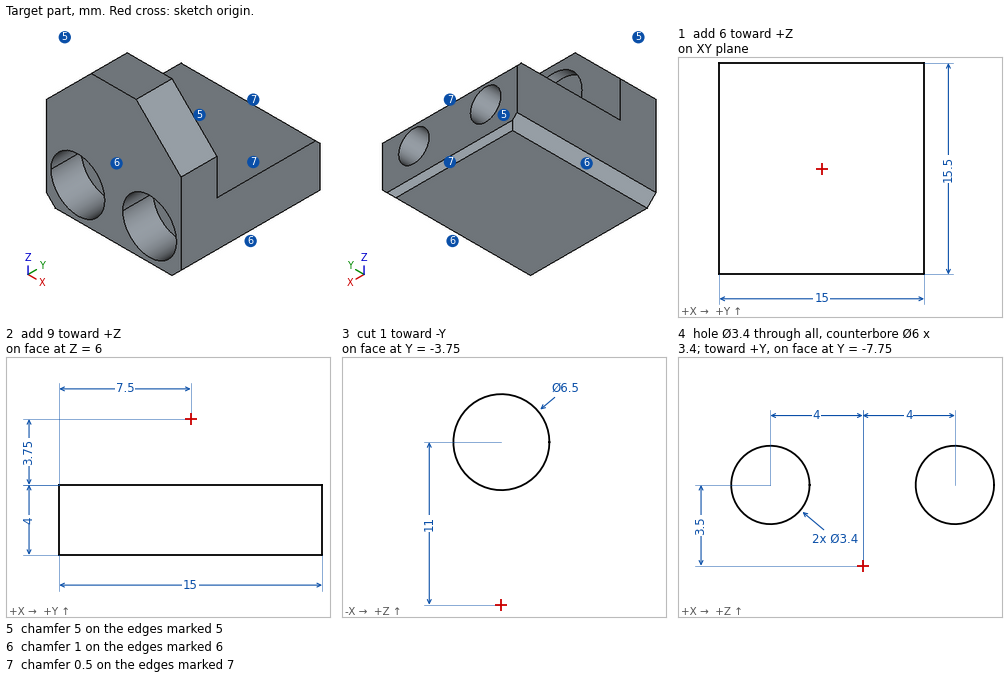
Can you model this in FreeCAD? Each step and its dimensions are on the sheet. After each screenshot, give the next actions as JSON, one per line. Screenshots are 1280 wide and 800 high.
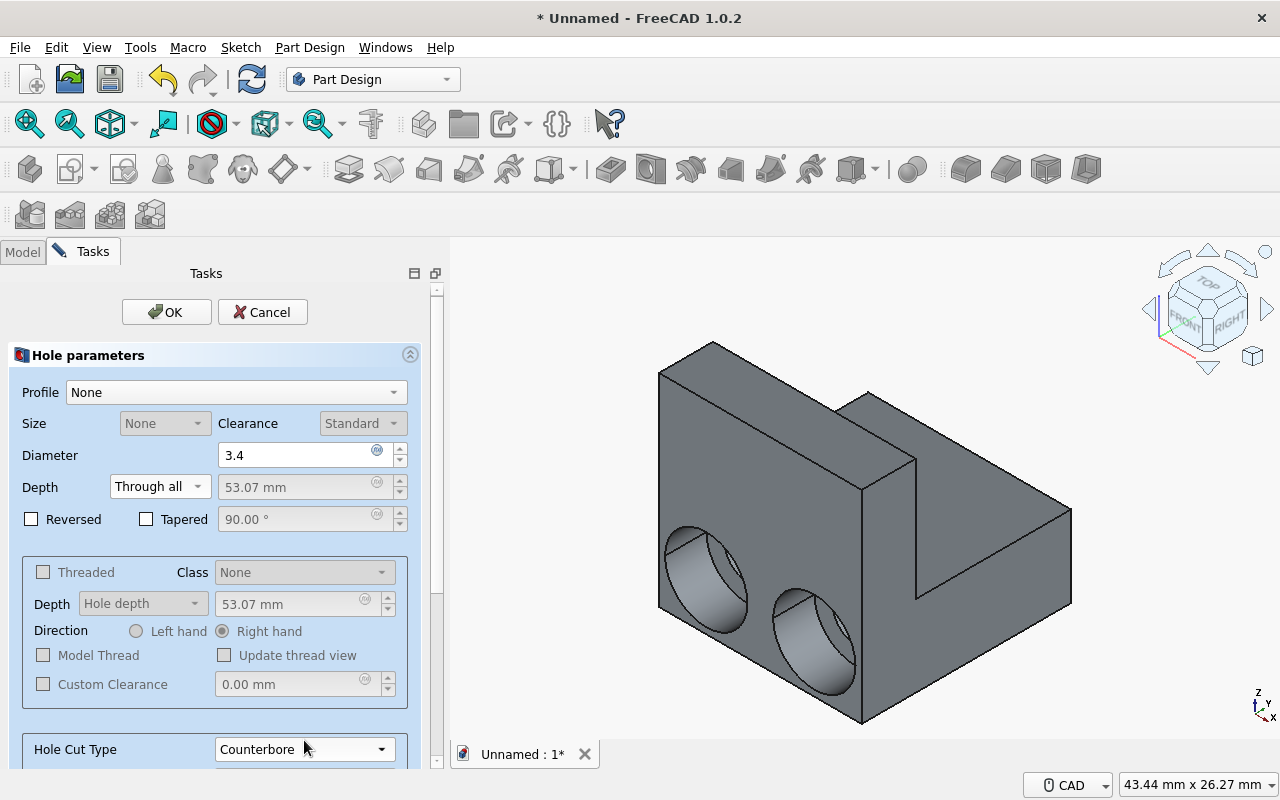
{"action": "scroll", "coordinate": [437, 526], "scroll_direction": "down", "scroll_amount": 2}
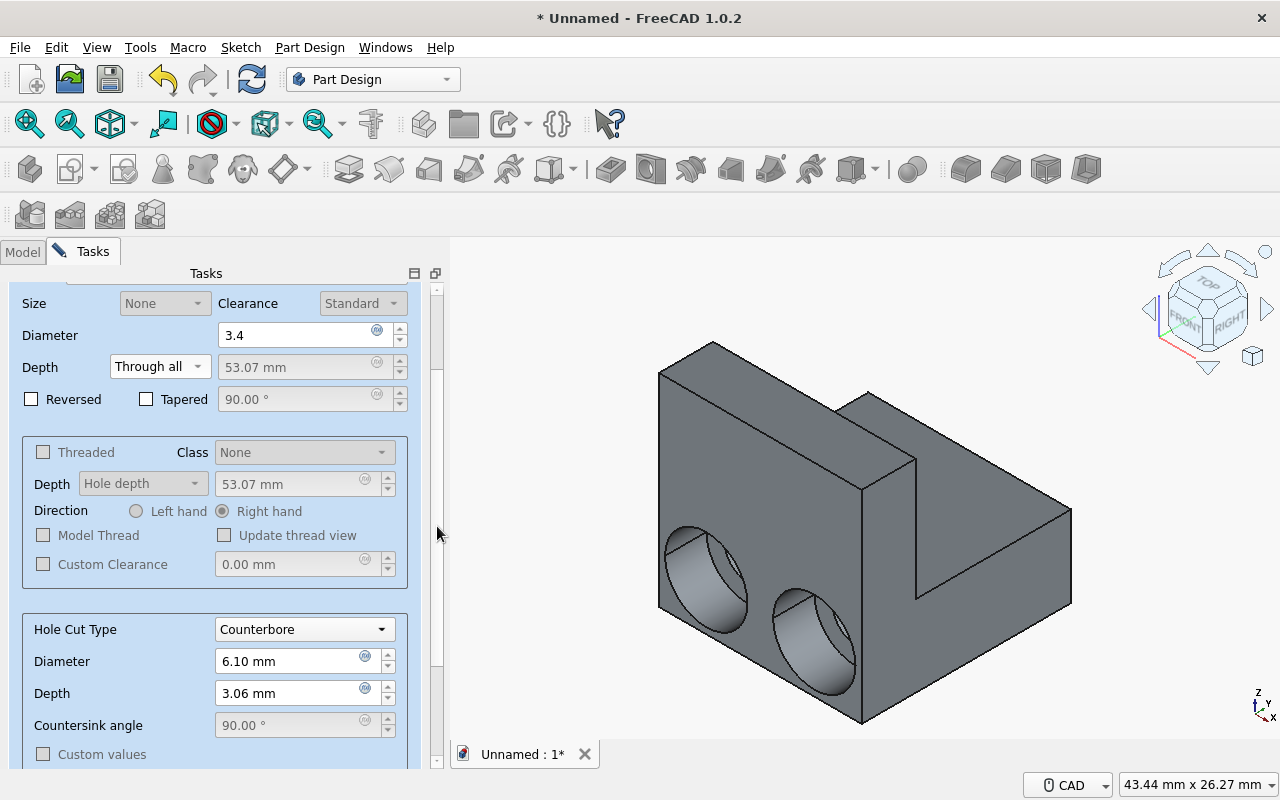
{"action": "triple_click", "coordinate": [298, 661]}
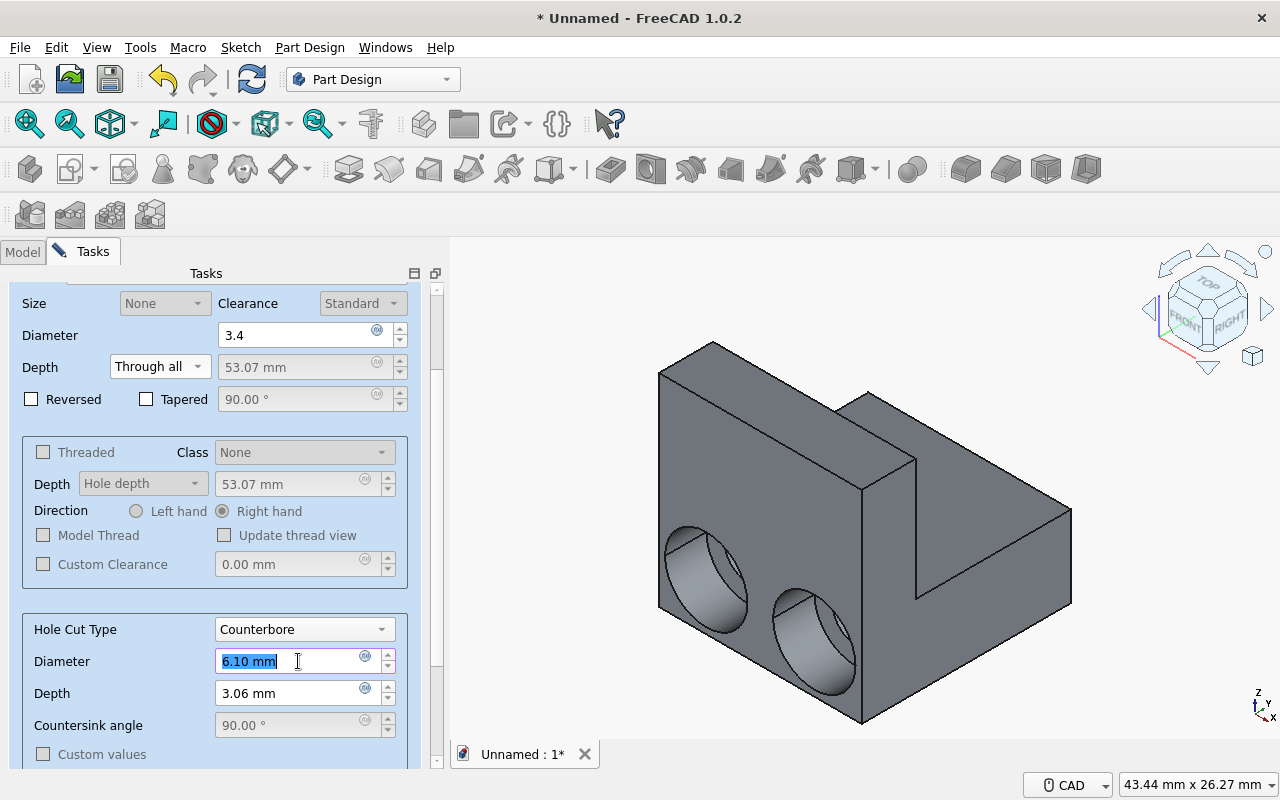
{"action": "type", "text": "6"}
{"action": "key", "text": "Tab"}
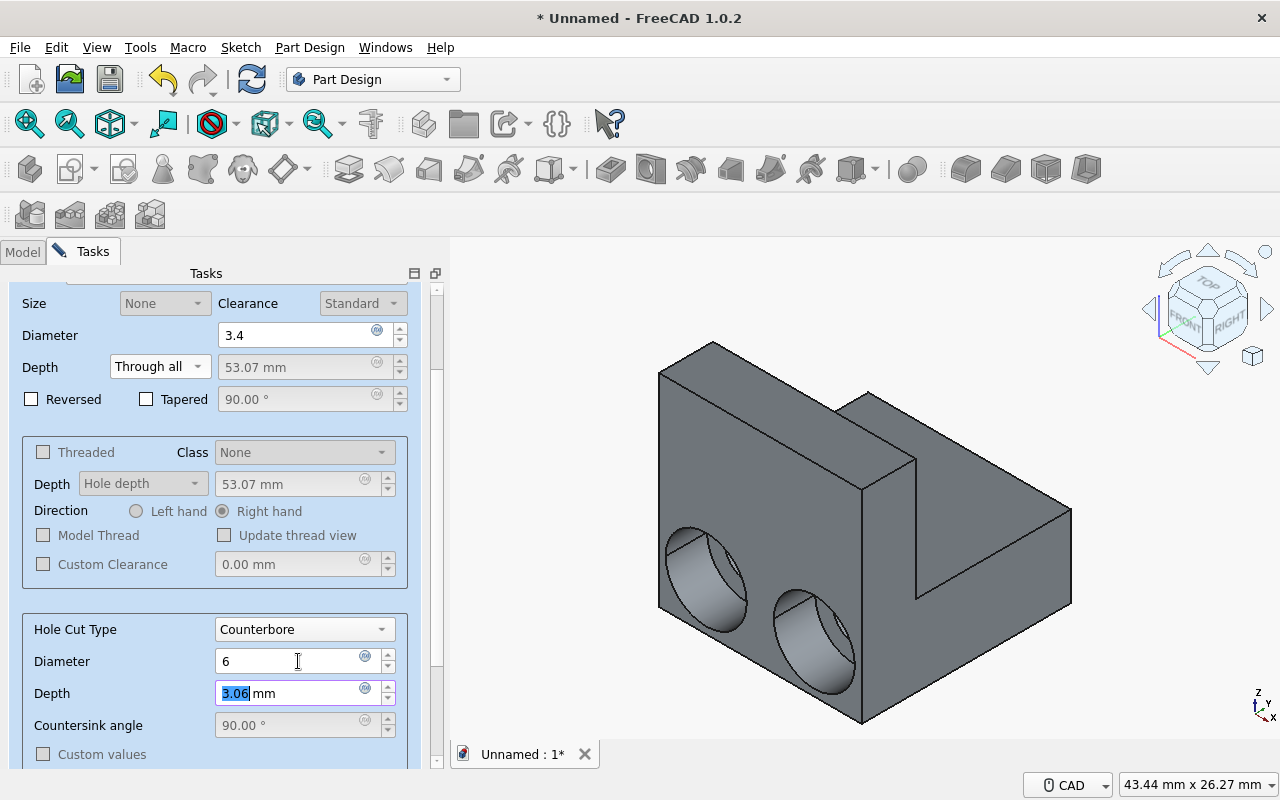
{"action": "type", "text": "3.4"}
{"action": "key", "text": "Tab"}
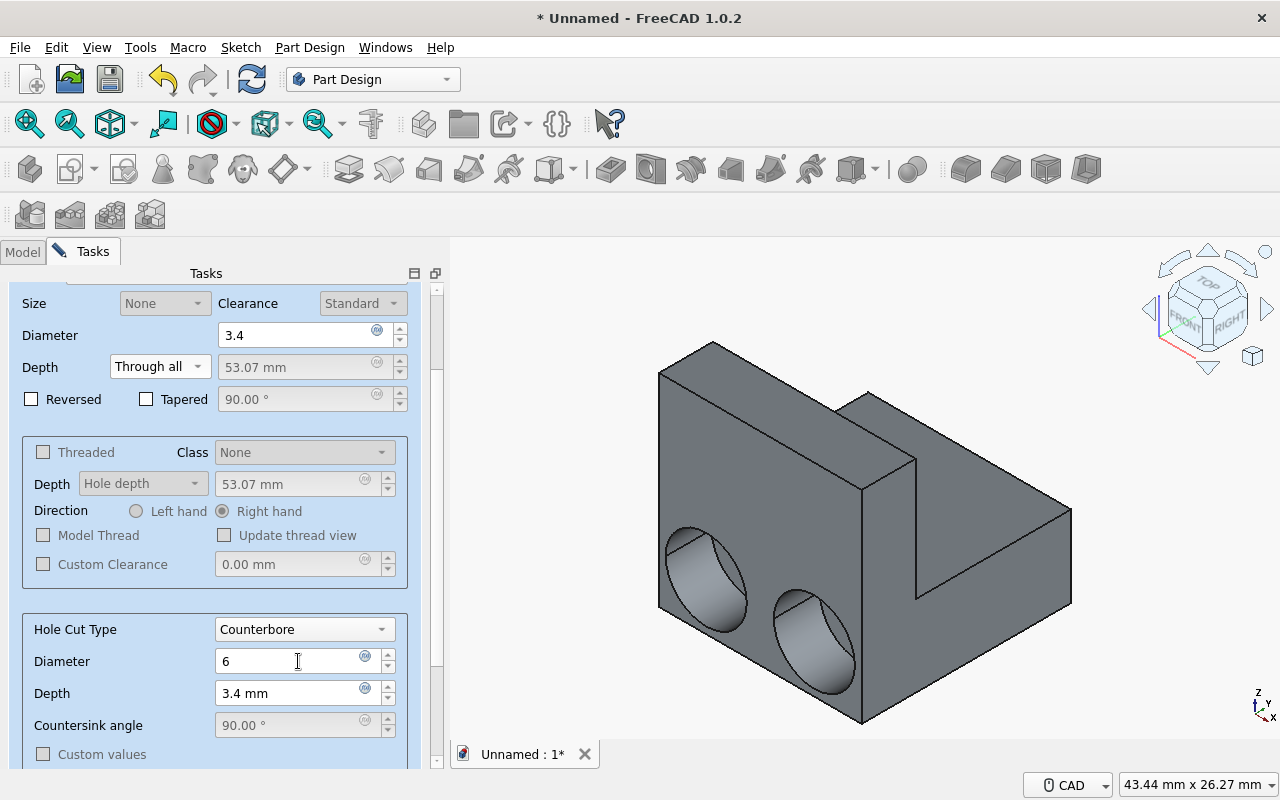
{"action": "scroll", "coordinate": [437, 526], "scroll_direction": "up", "scroll_amount": 3}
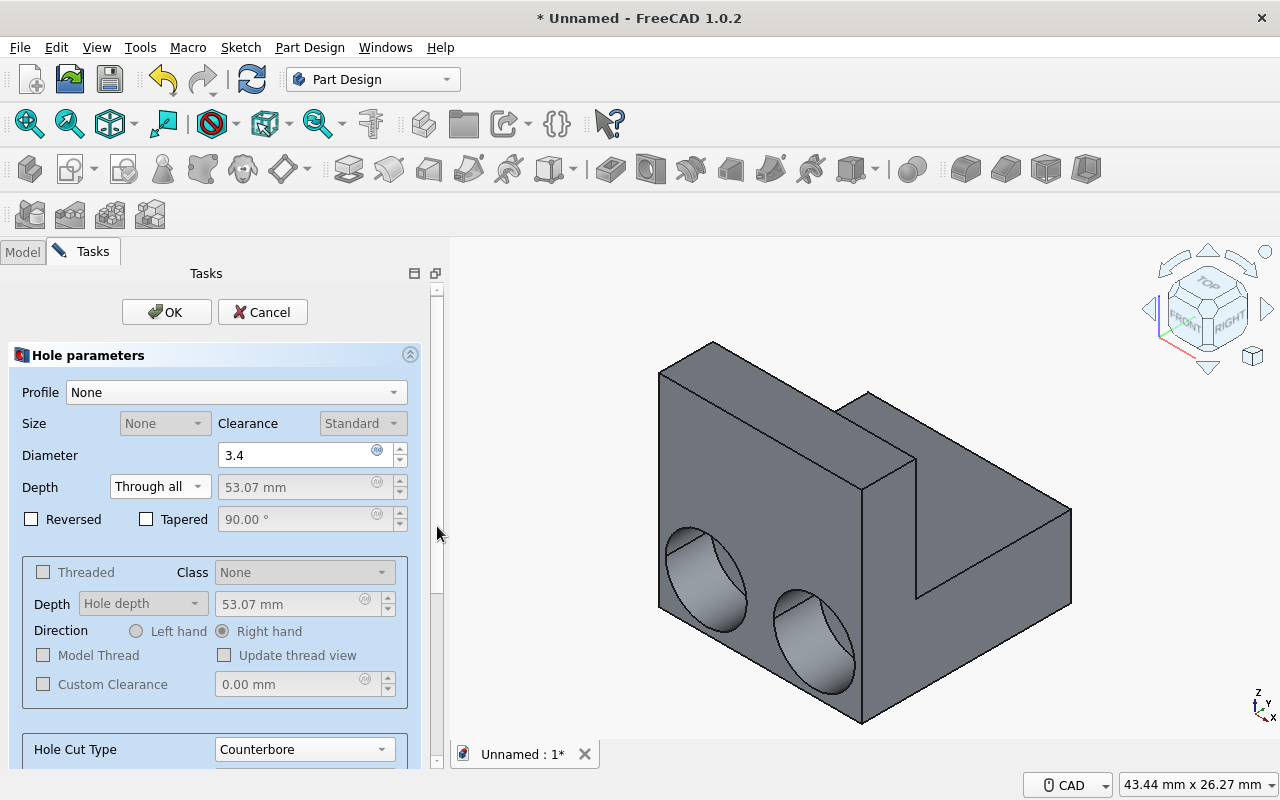
{"action": "left_click", "coordinate": [167, 312]}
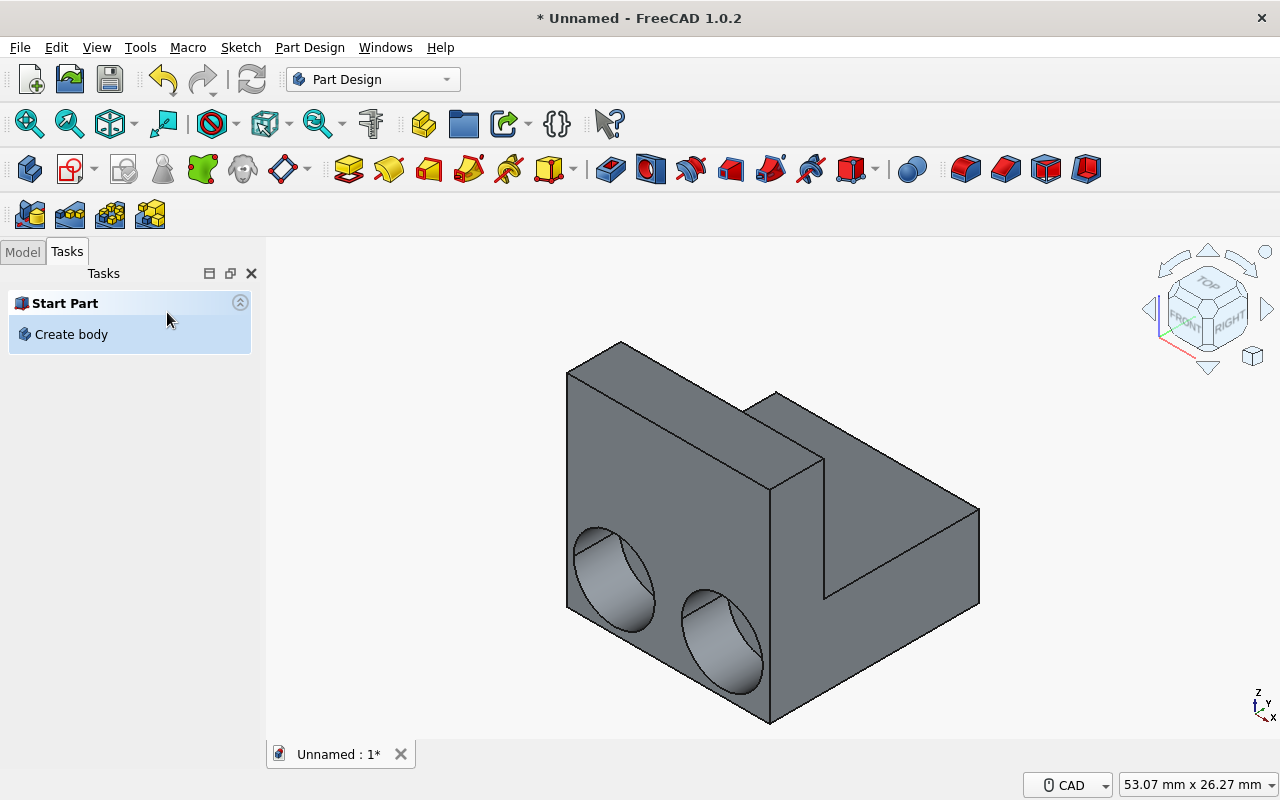
{"action": "left_click", "coordinate": [797, 473]}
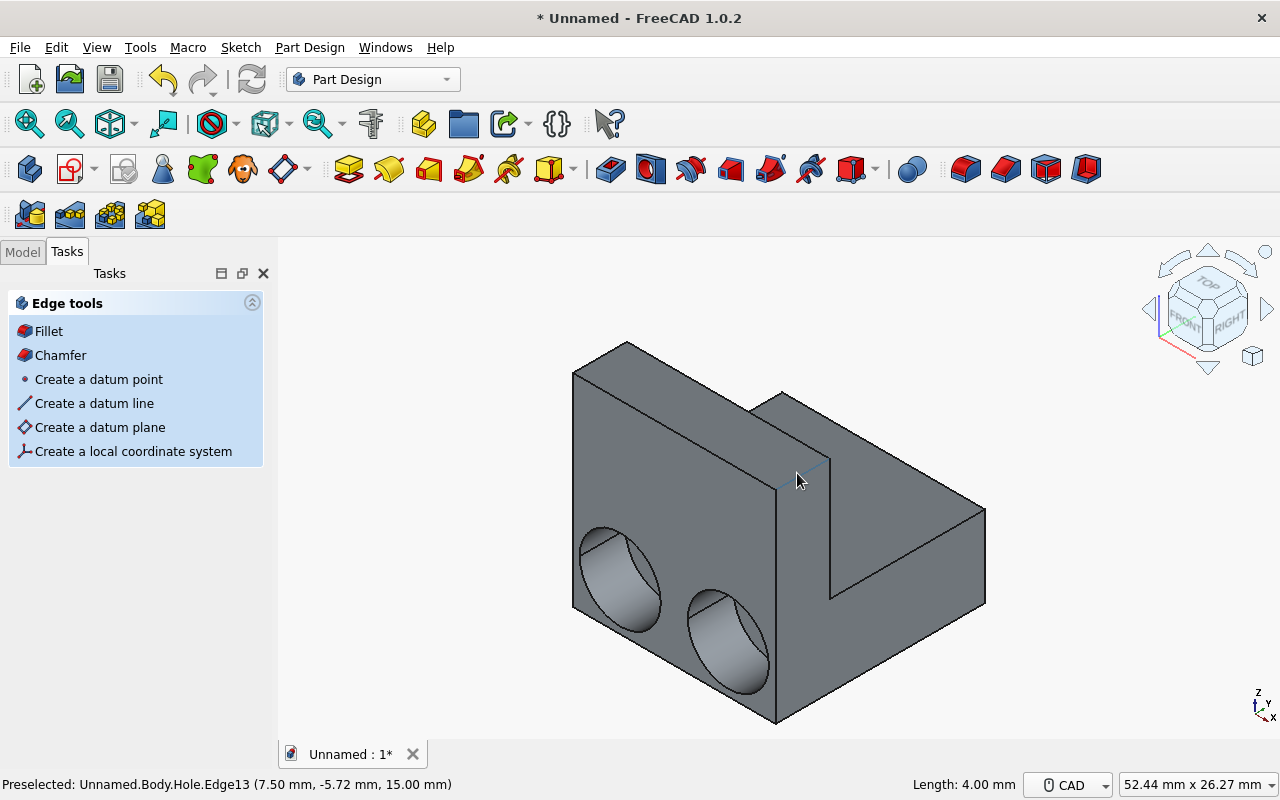
{"action": "key", "text": "2"}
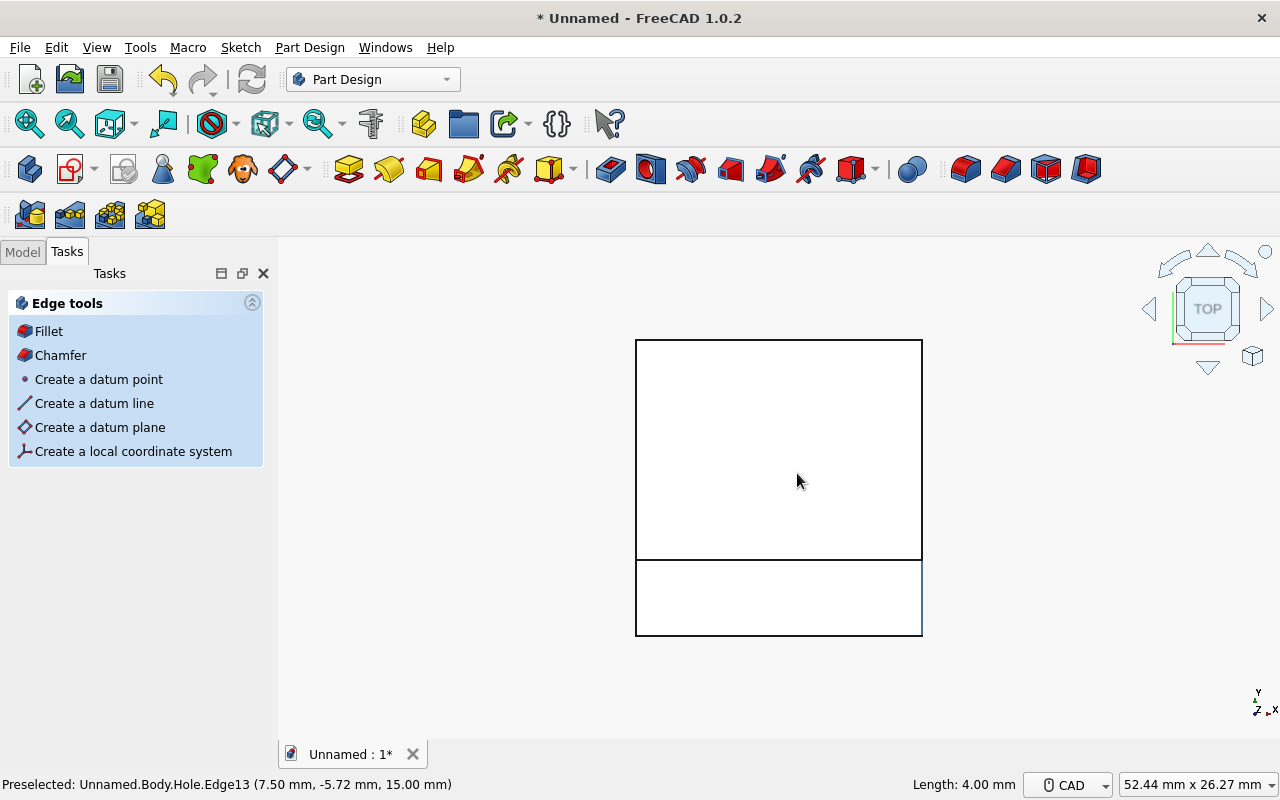
{"action": "left_click", "coordinate": [636, 597], "text": "ctrl"}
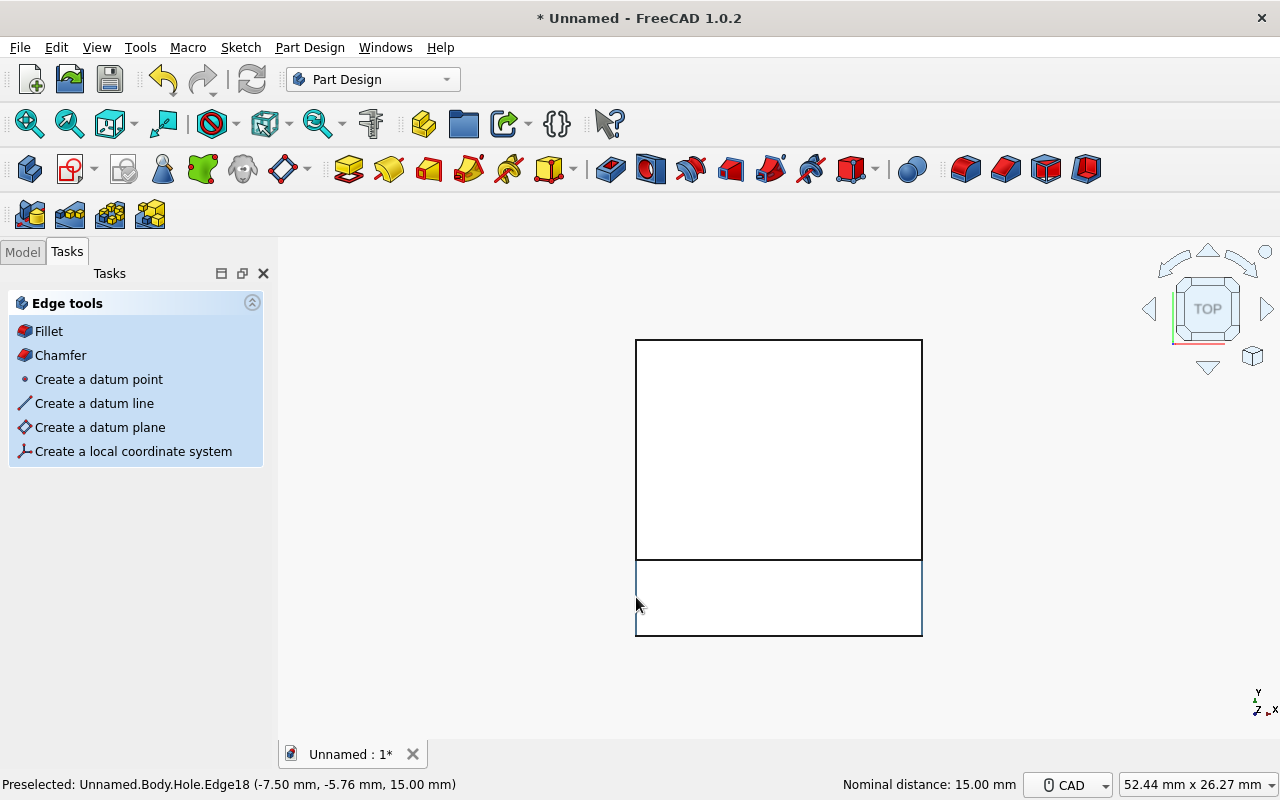
{"action": "left_click", "coordinate": [1006, 170]}